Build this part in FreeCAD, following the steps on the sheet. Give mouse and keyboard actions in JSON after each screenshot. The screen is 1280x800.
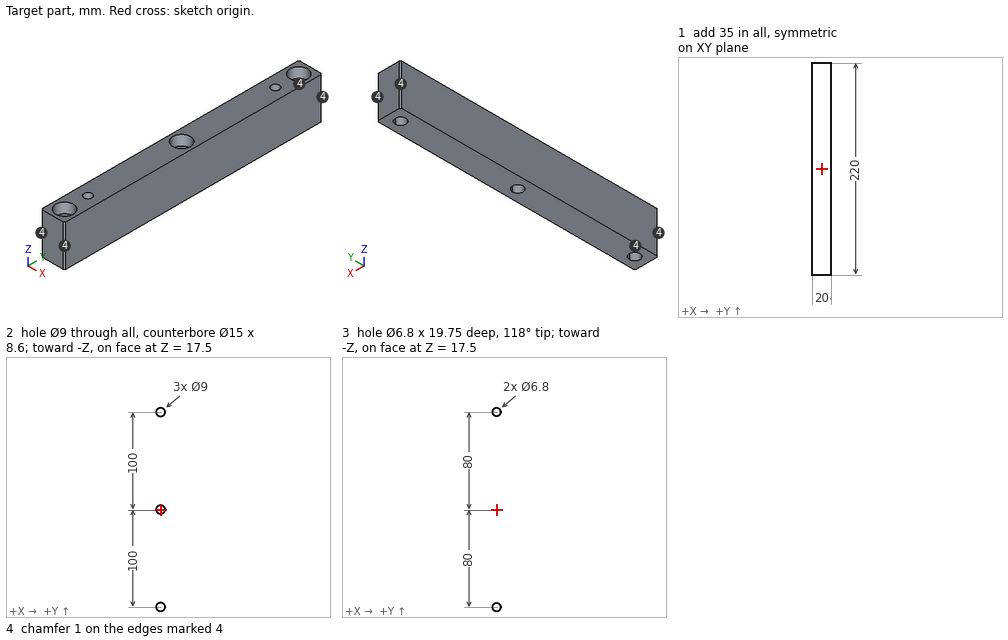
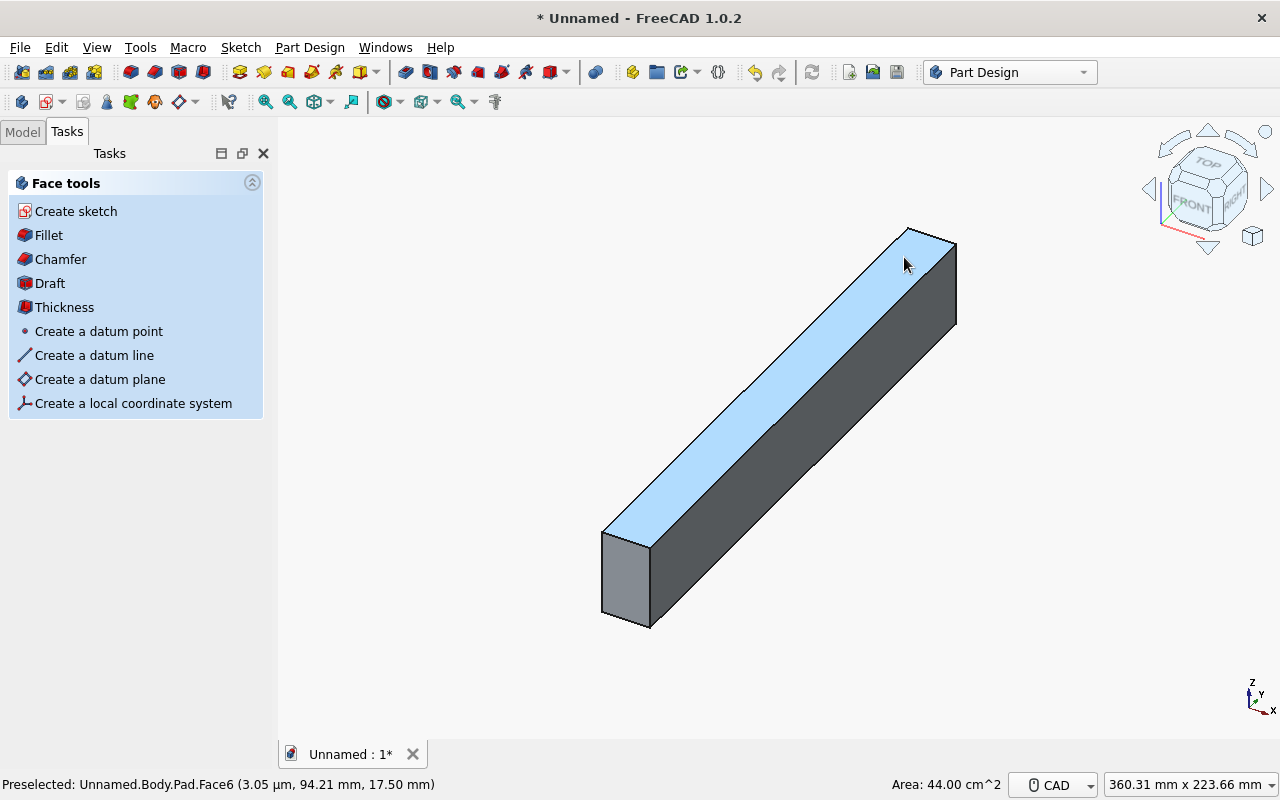
{"action": "left_click", "coordinate": [46, 102]}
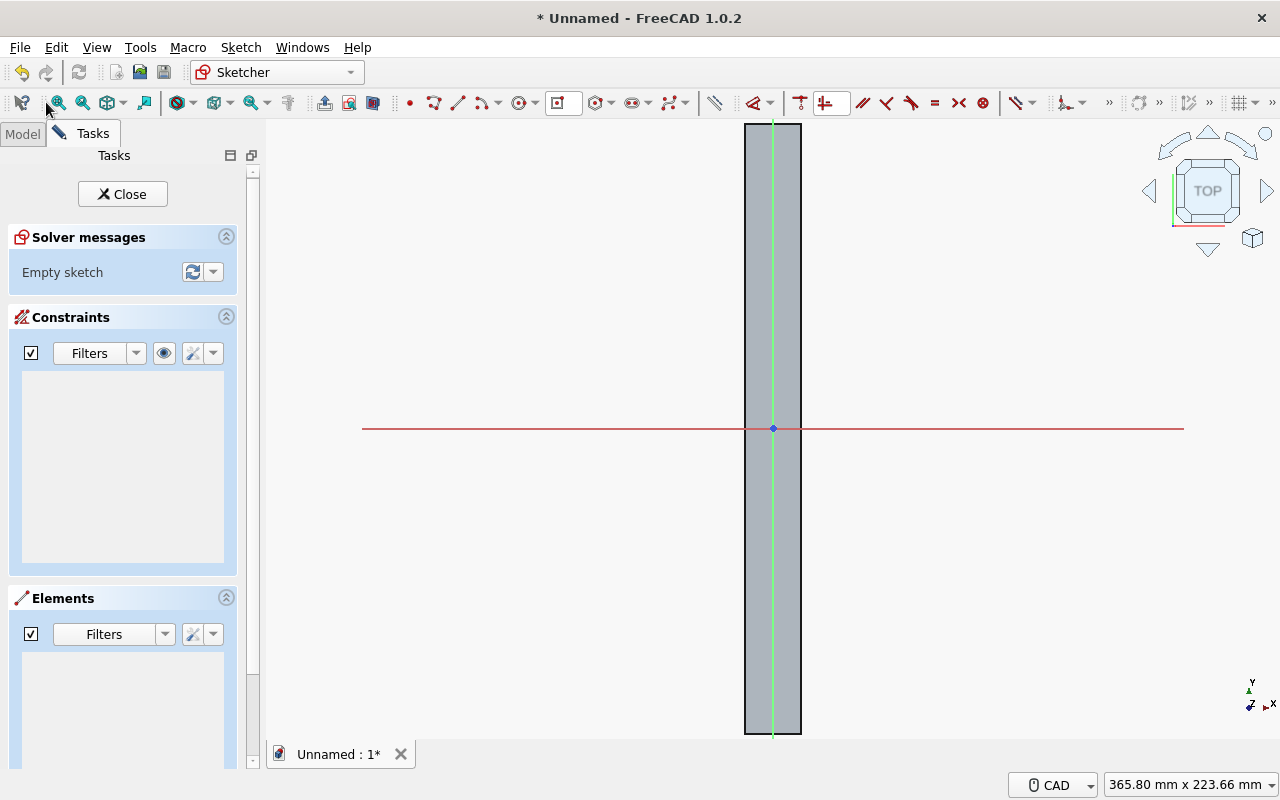
{"action": "scroll", "coordinate": [565, 429], "scroll_direction": "down", "scroll_amount": 2}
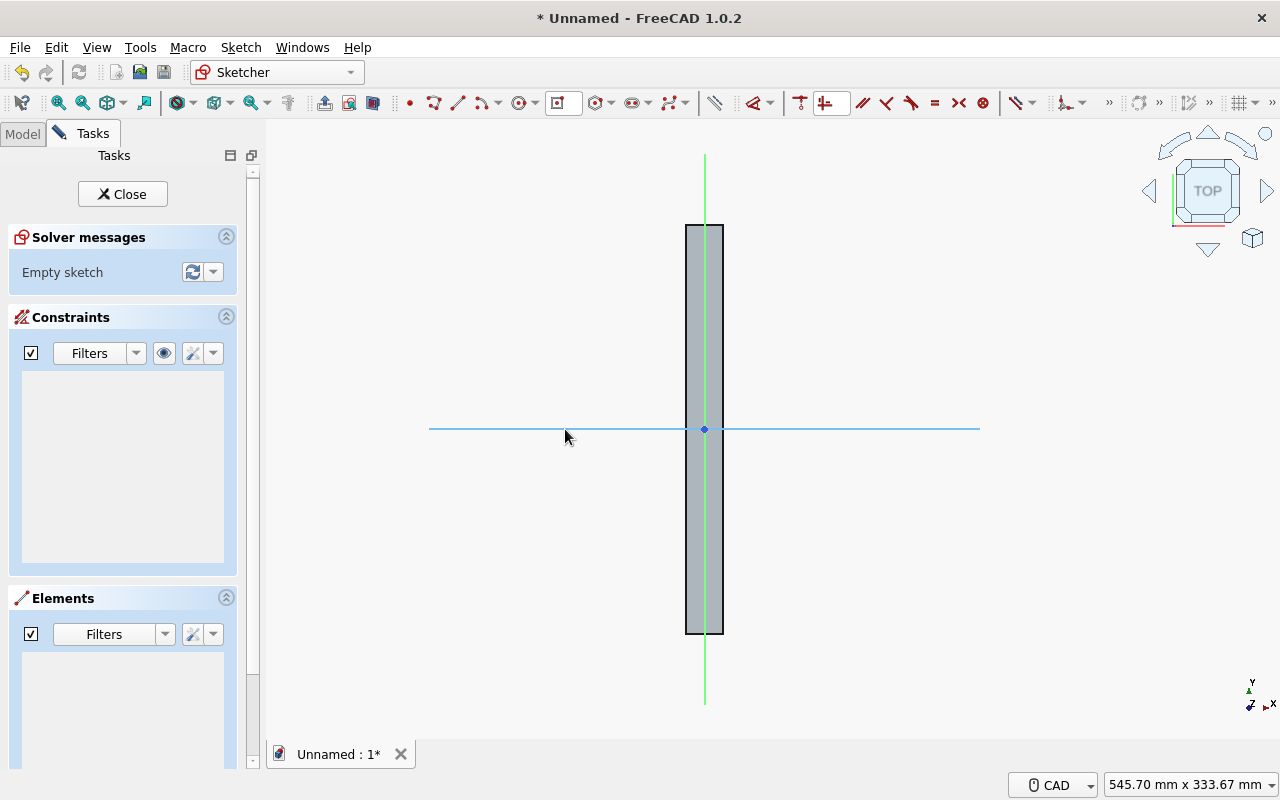
{"action": "left_click", "coordinate": [520, 104]}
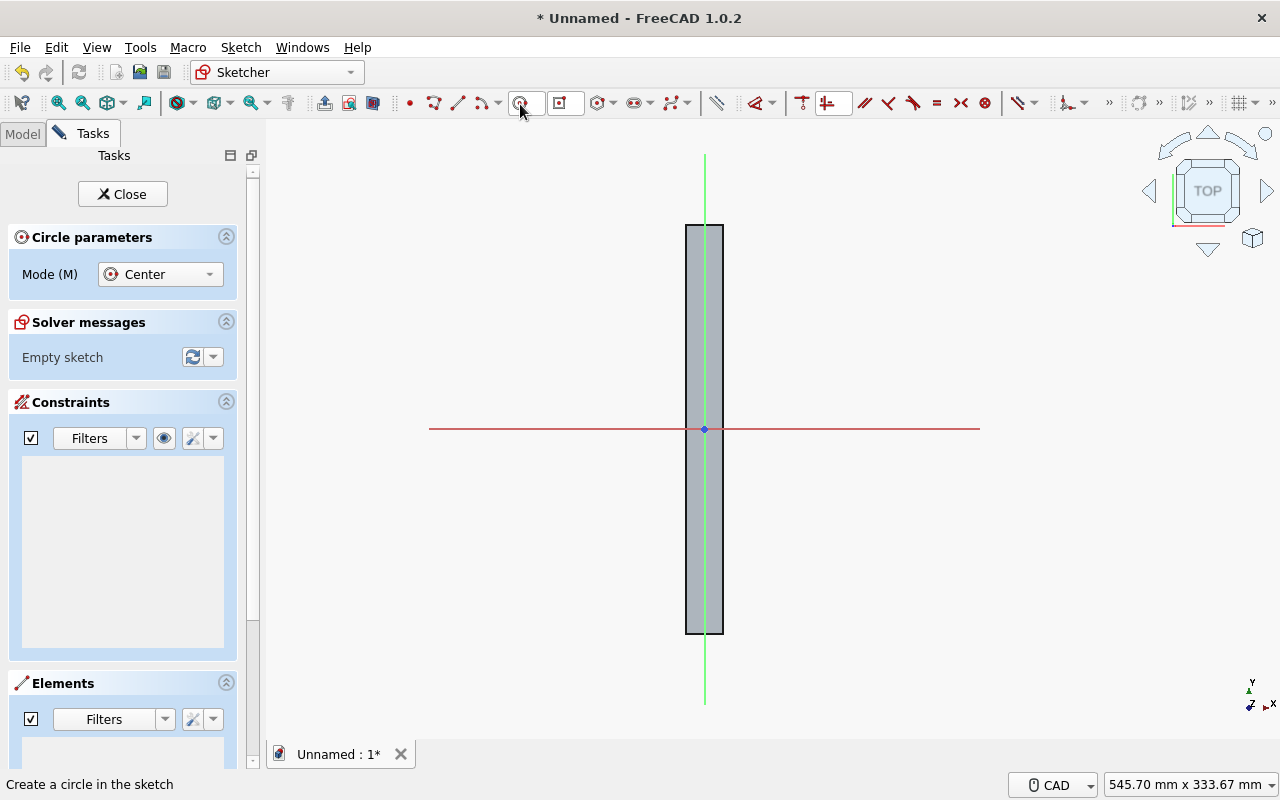
{"action": "scroll", "coordinate": [705, 243], "scroll_direction": "up", "scroll_amount": 5}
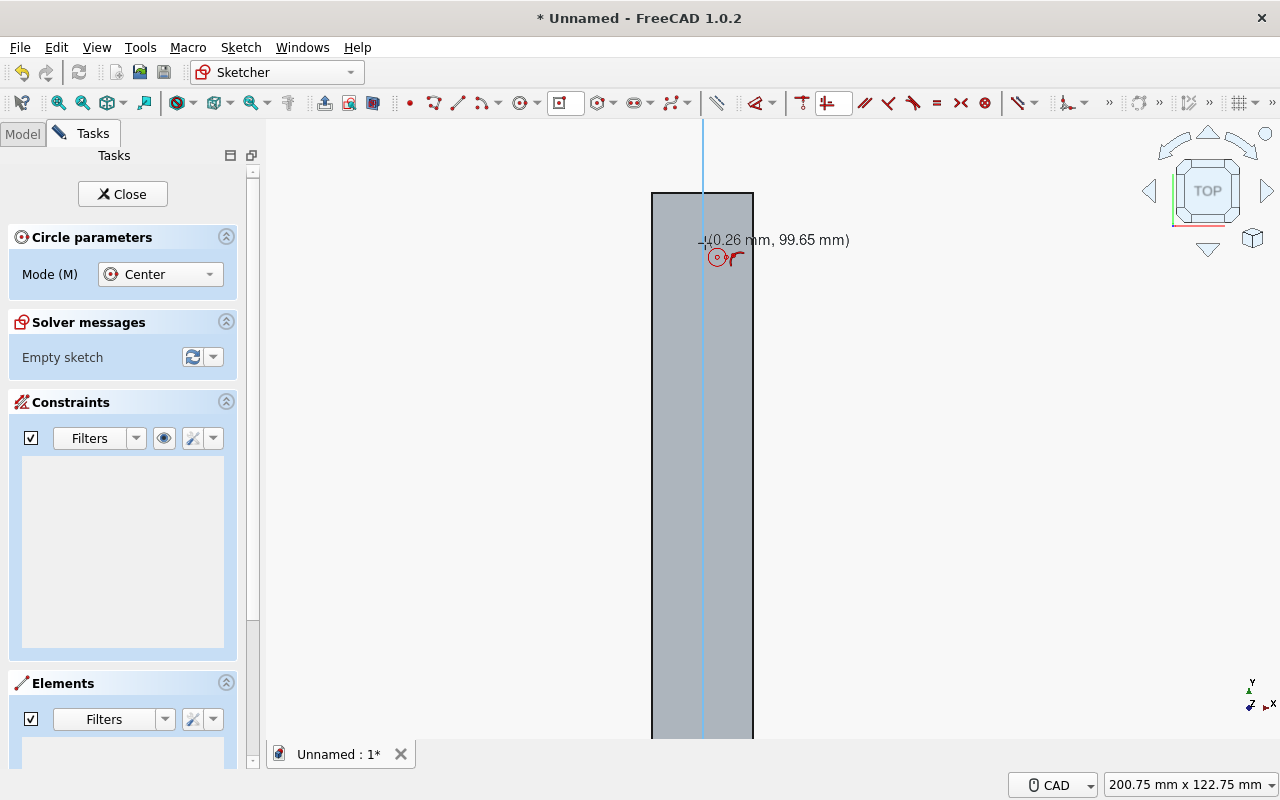
{"action": "left_click", "coordinate": [703, 244]}
{"action": "left_click", "coordinate": [719, 228]}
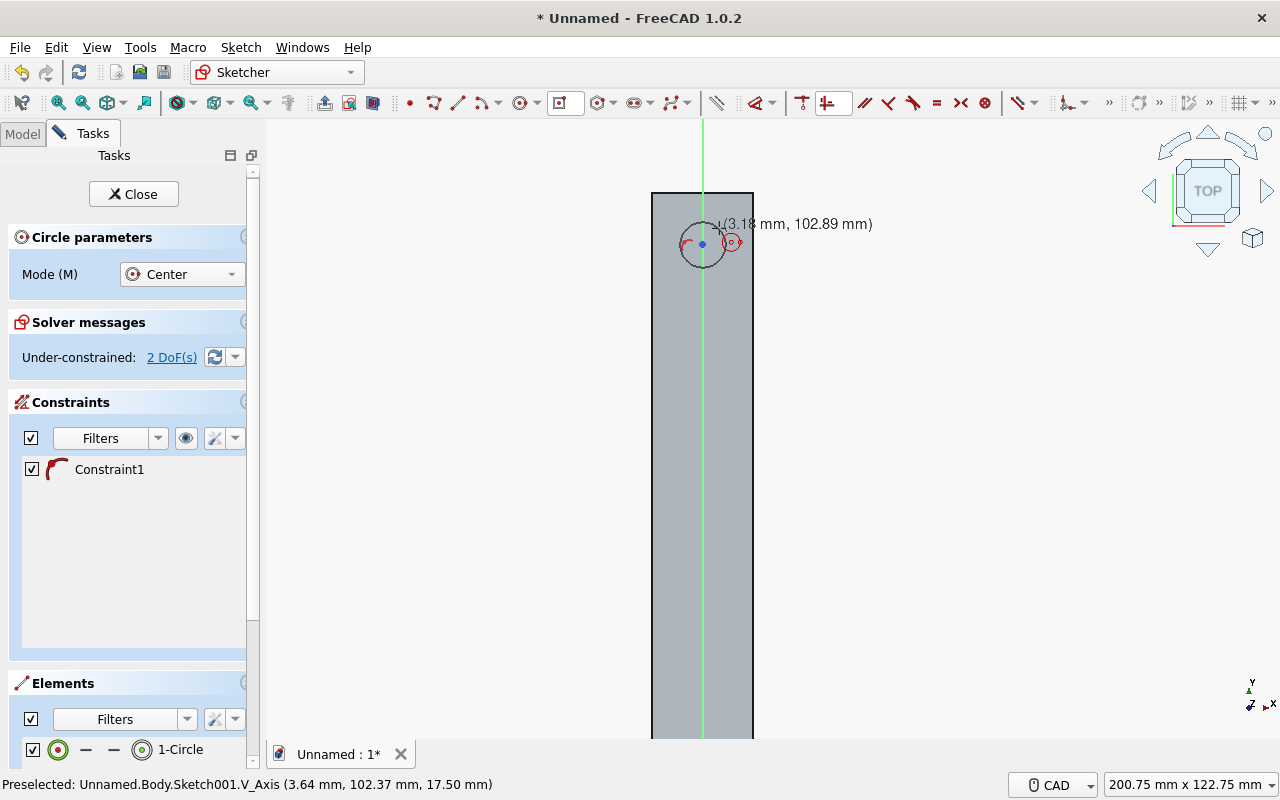
{"action": "scroll", "coordinate": [705, 243], "scroll_direction": "down", "scroll_amount": 5}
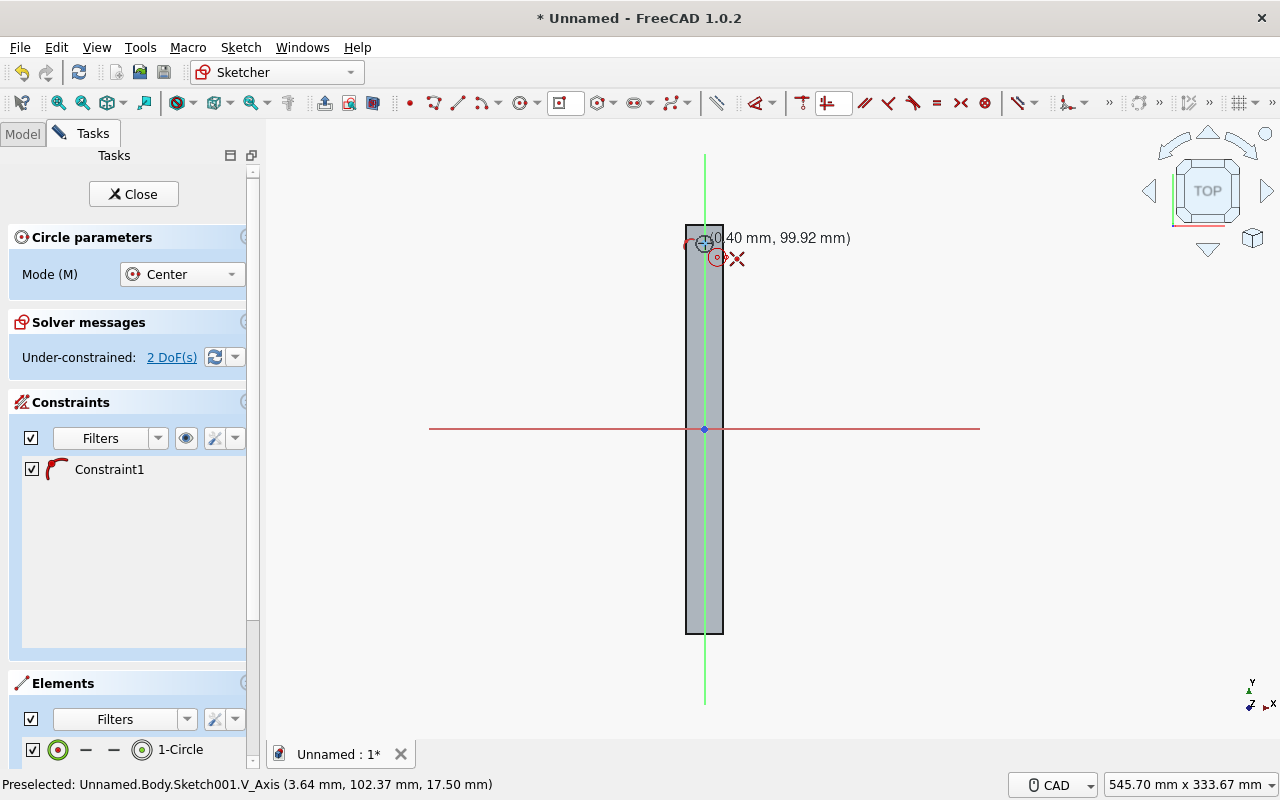
{"action": "scroll", "coordinate": [705, 429], "scroll_direction": "up", "scroll_amount": 5}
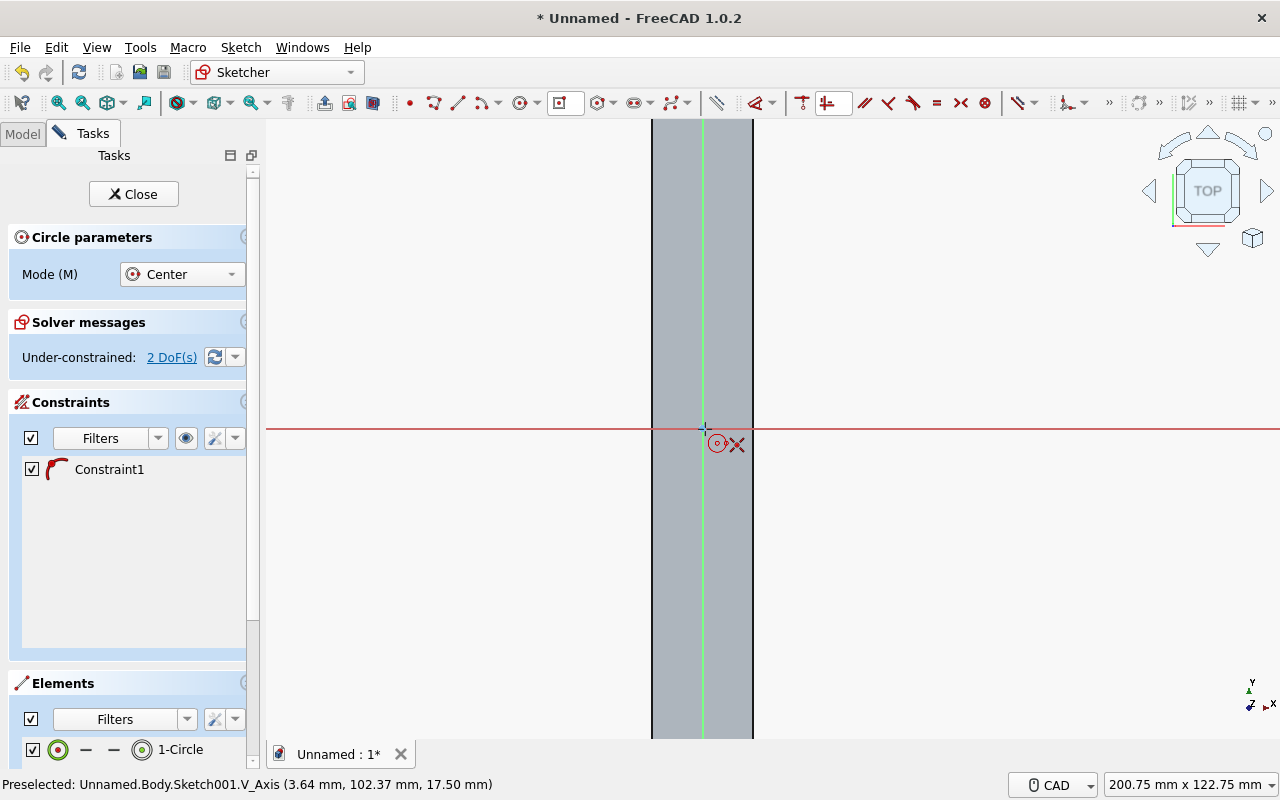
{"action": "left_click", "coordinate": [703, 429]}
{"action": "left_click", "coordinate": [719, 413]}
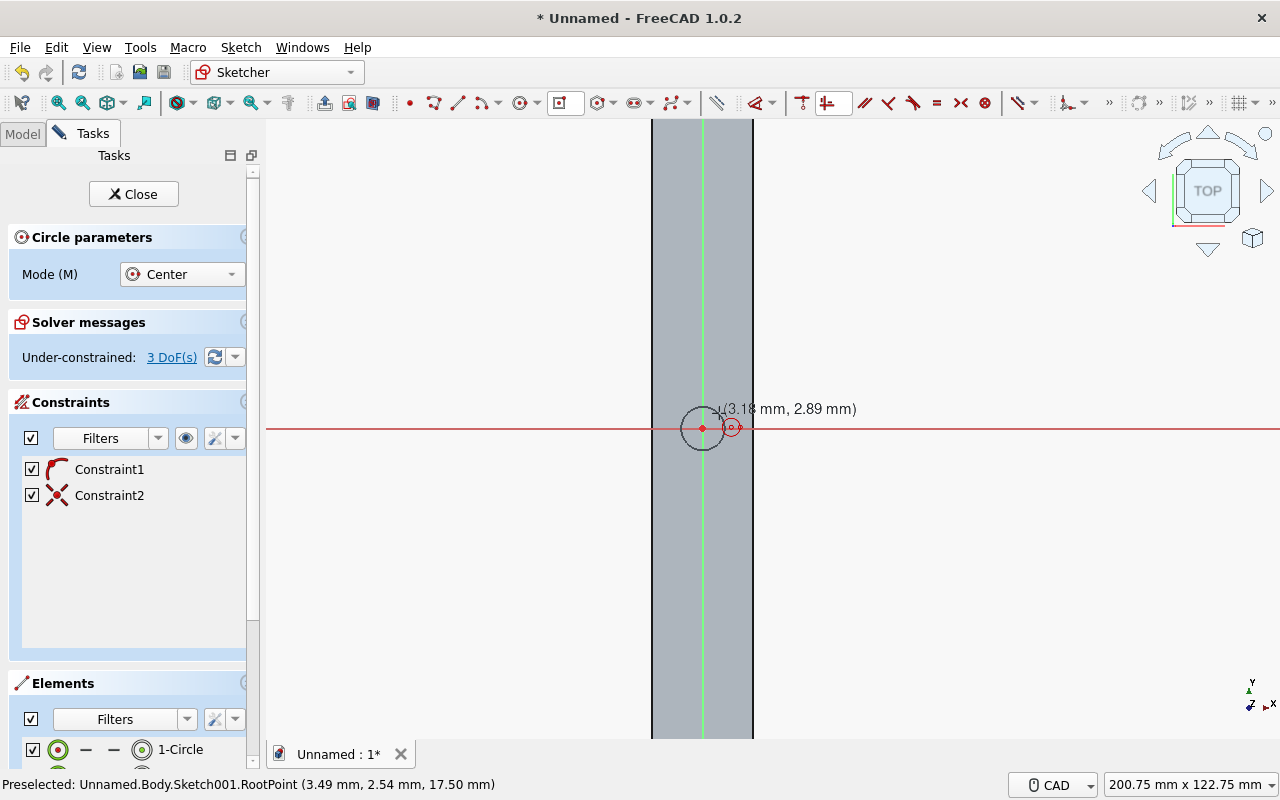
{"action": "scroll", "coordinate": [705, 429], "scroll_direction": "down", "scroll_amount": 5}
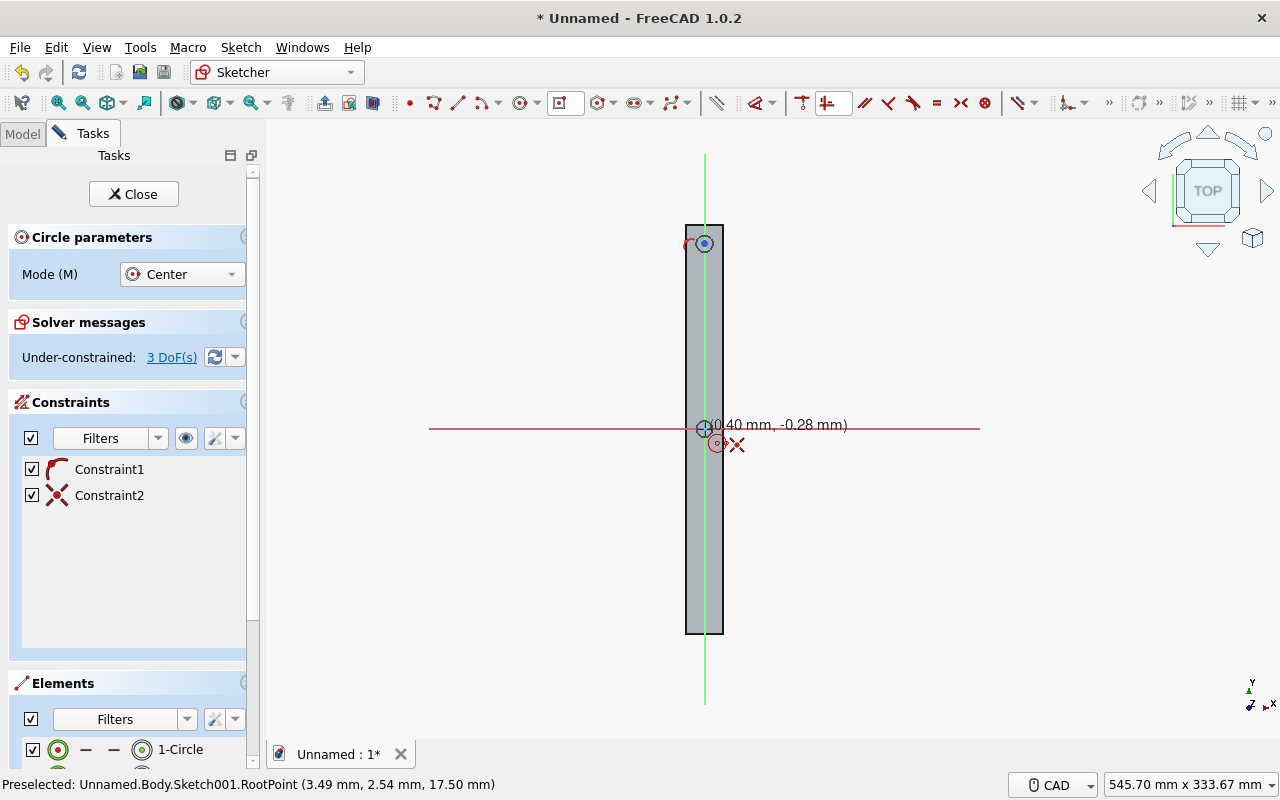
{"action": "scroll", "coordinate": [705, 615], "scroll_direction": "up", "scroll_amount": 5}